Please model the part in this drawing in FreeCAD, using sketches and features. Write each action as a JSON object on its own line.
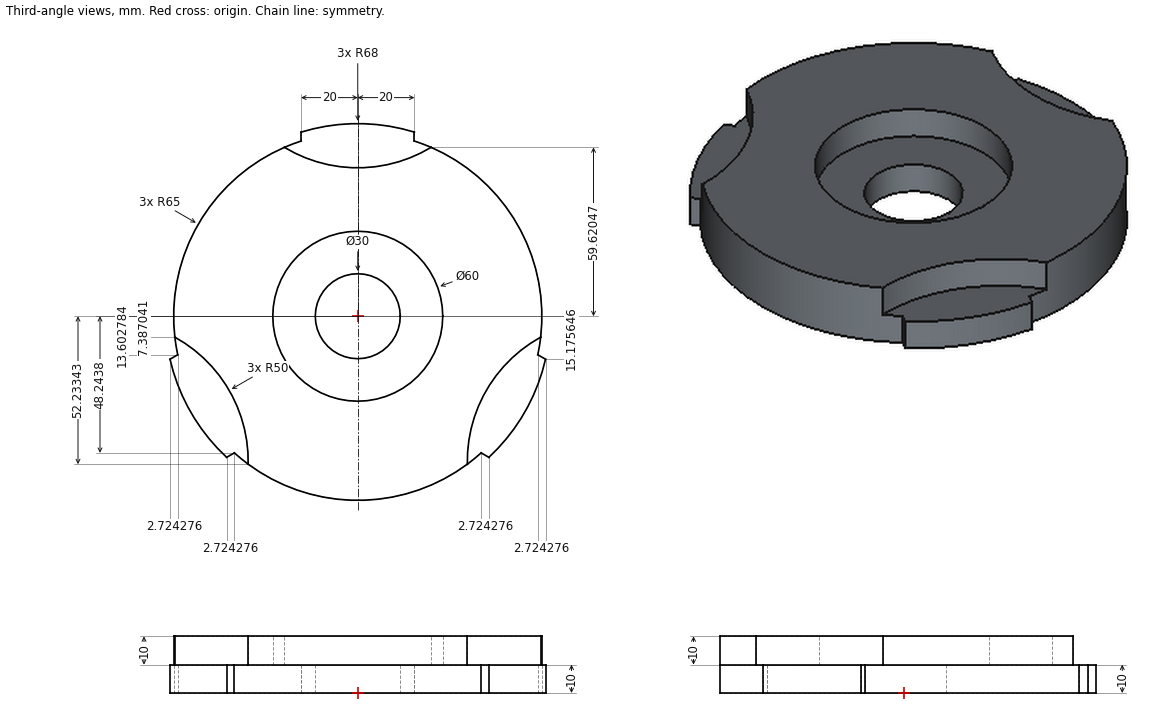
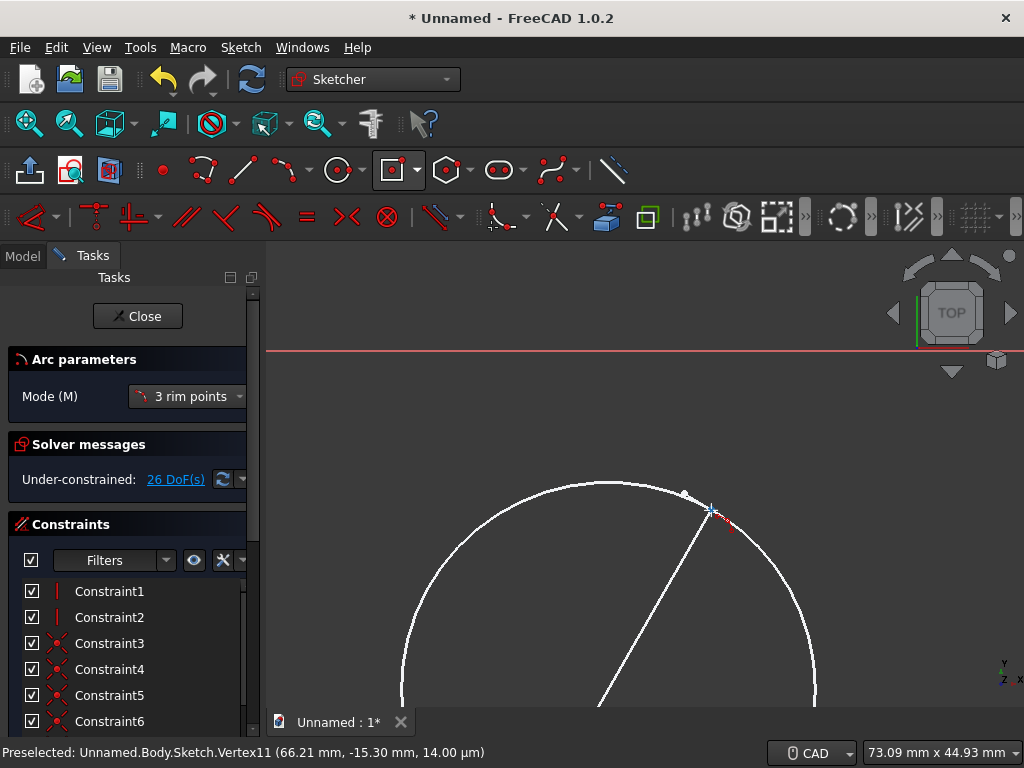
{"action": "scroll", "coordinate": [716, 509], "scroll_direction": "down", "scroll_amount": 8}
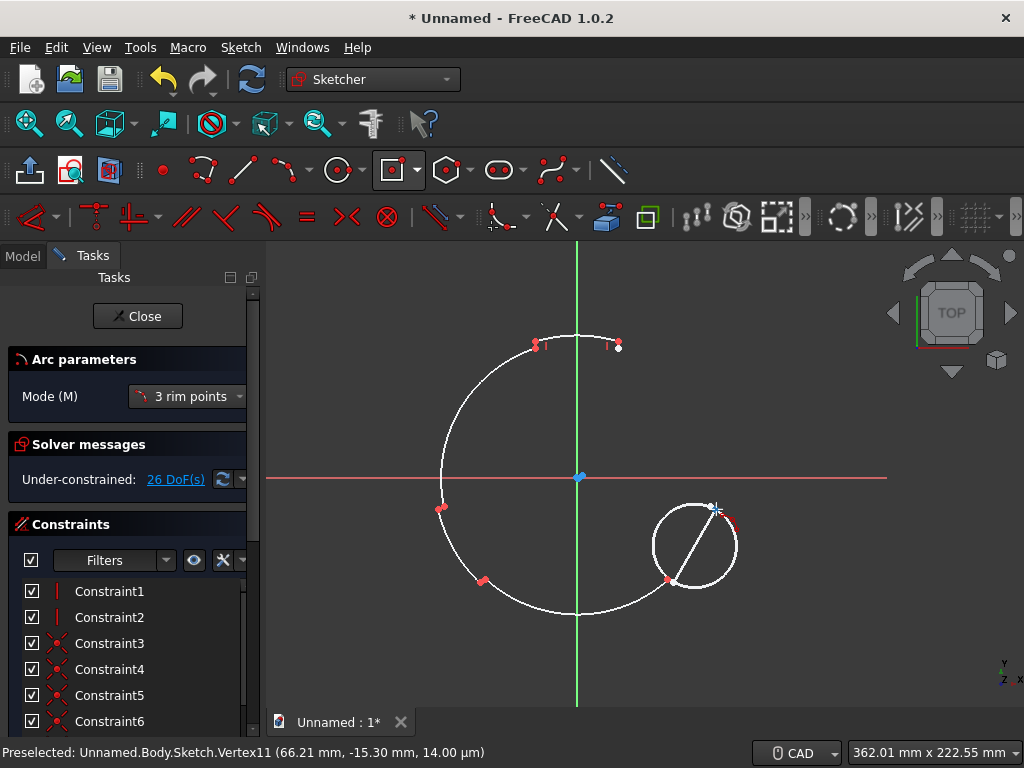
{"action": "scroll", "coordinate": [700, 549], "scroll_direction": "up", "scroll_amount": 5}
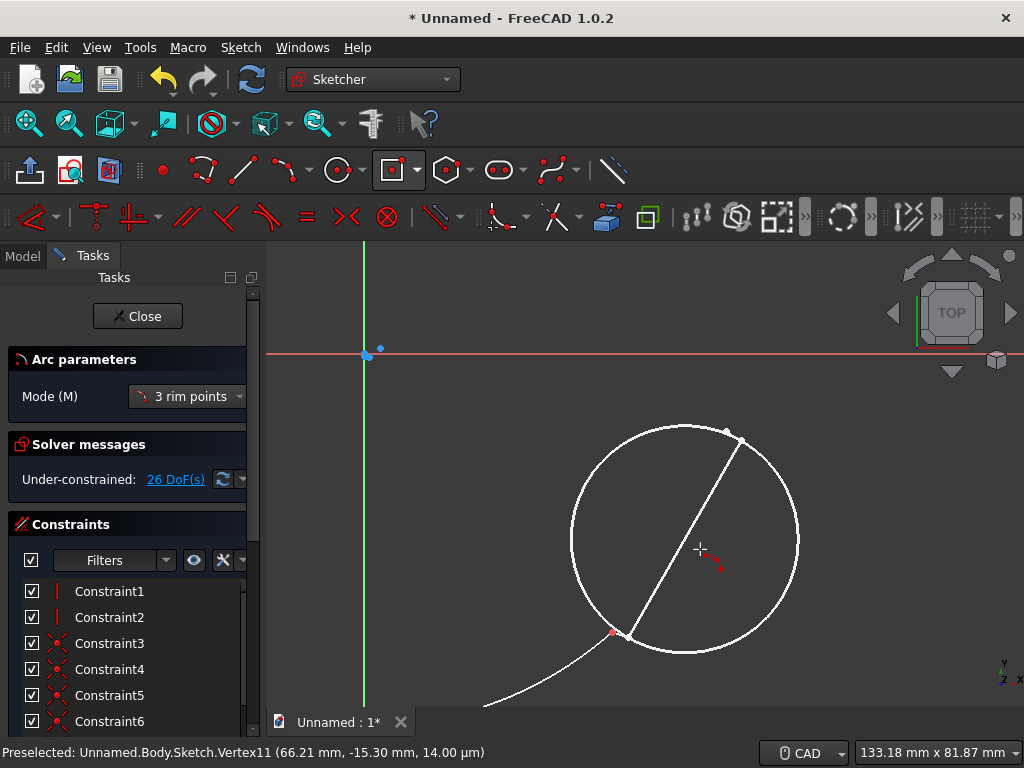
{"action": "left_click", "coordinate": [700, 547]}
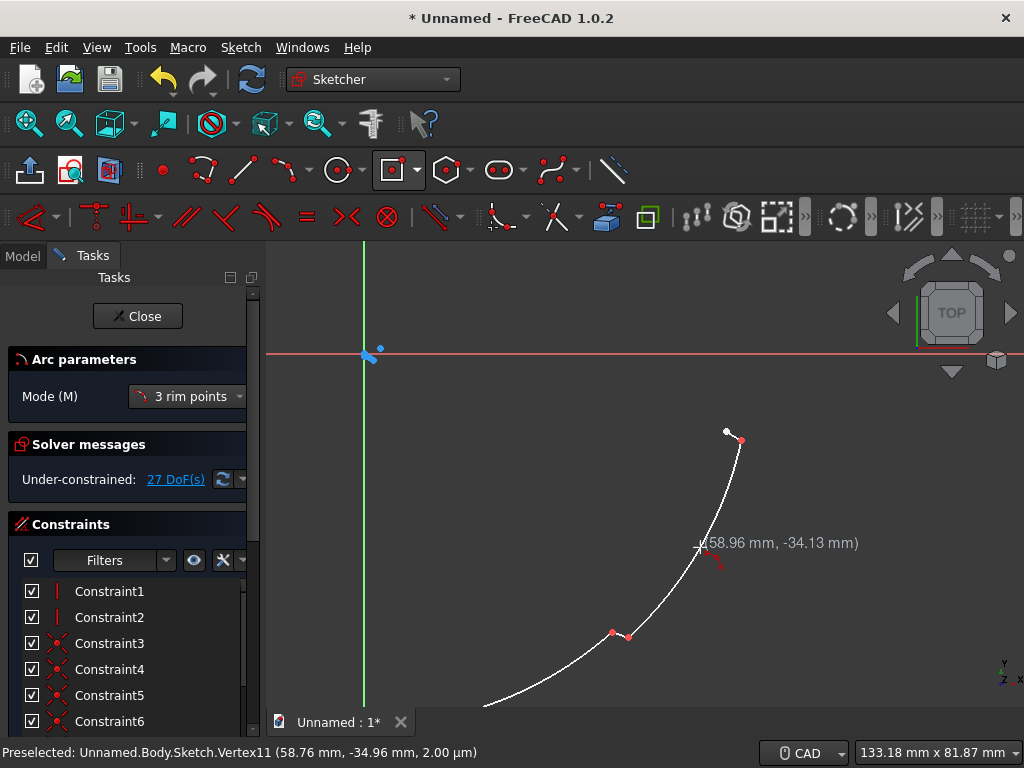
{"action": "scroll", "coordinate": [726, 431], "scroll_direction": "up", "scroll_amount": 3}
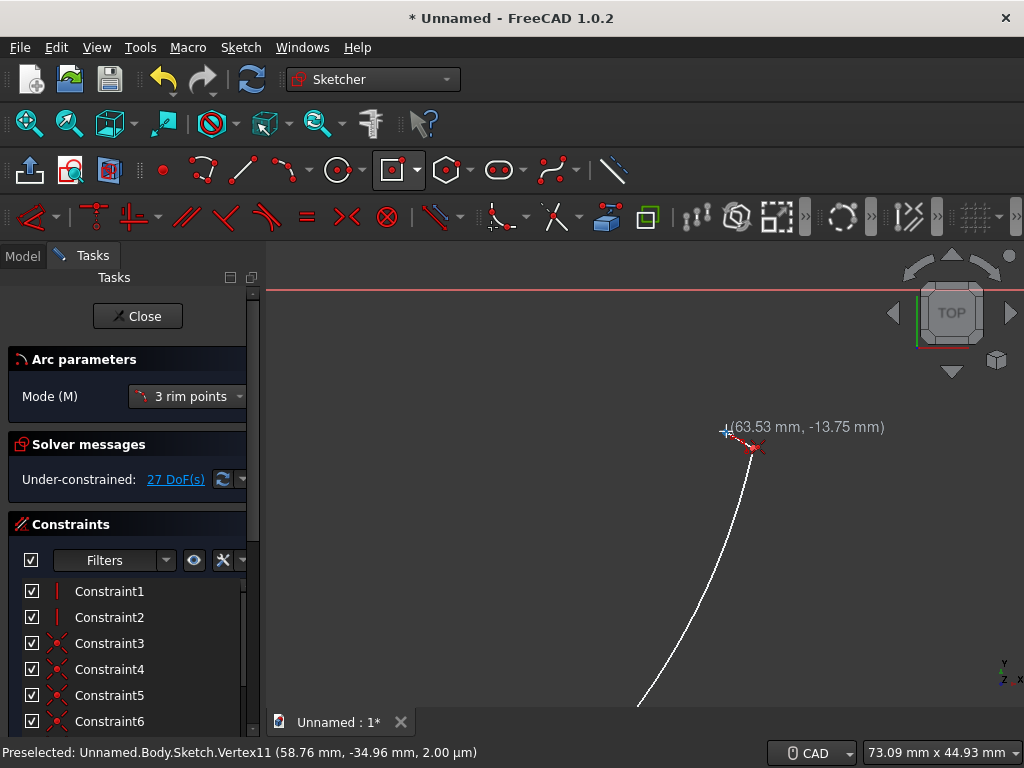
{"action": "left_click", "coordinate": [726, 432]}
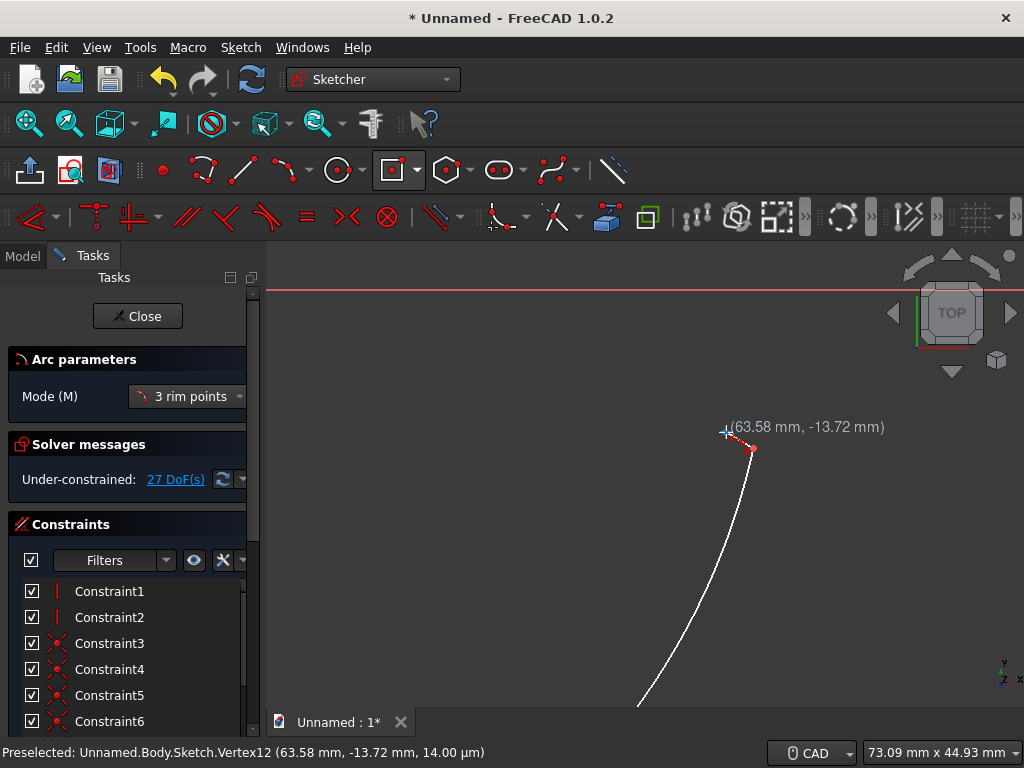
{"action": "scroll", "coordinate": [705, 525], "scroll_direction": "down", "scroll_amount": 8}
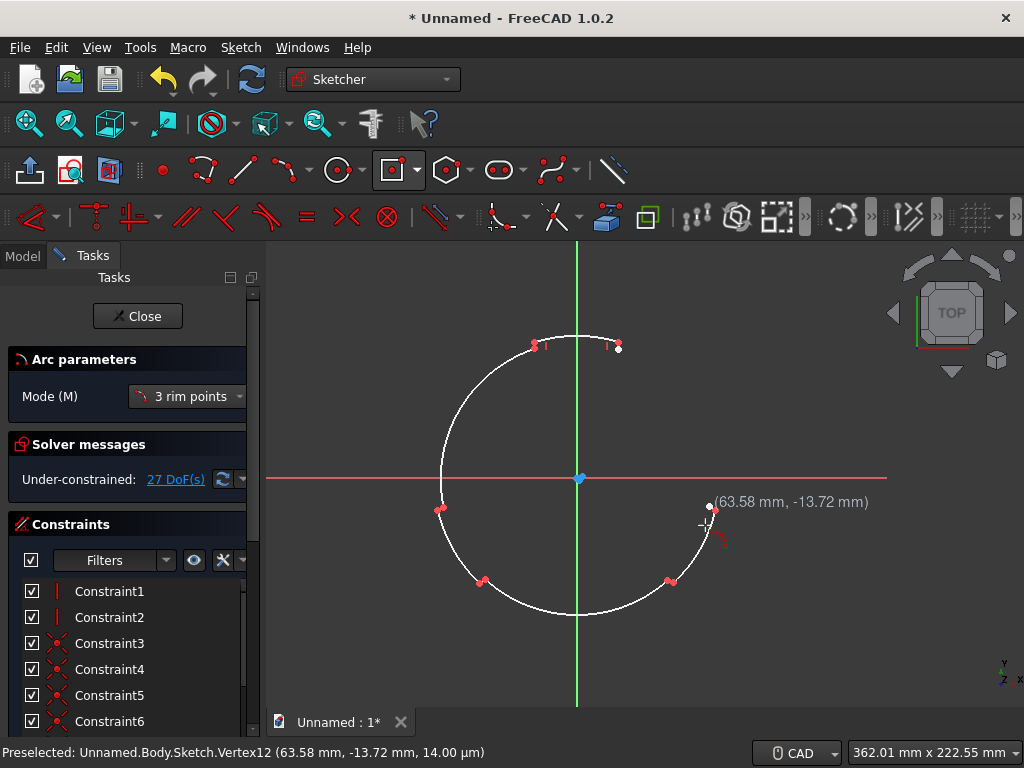
{"action": "scroll", "coordinate": [618, 349], "scroll_direction": "up", "scroll_amount": 8}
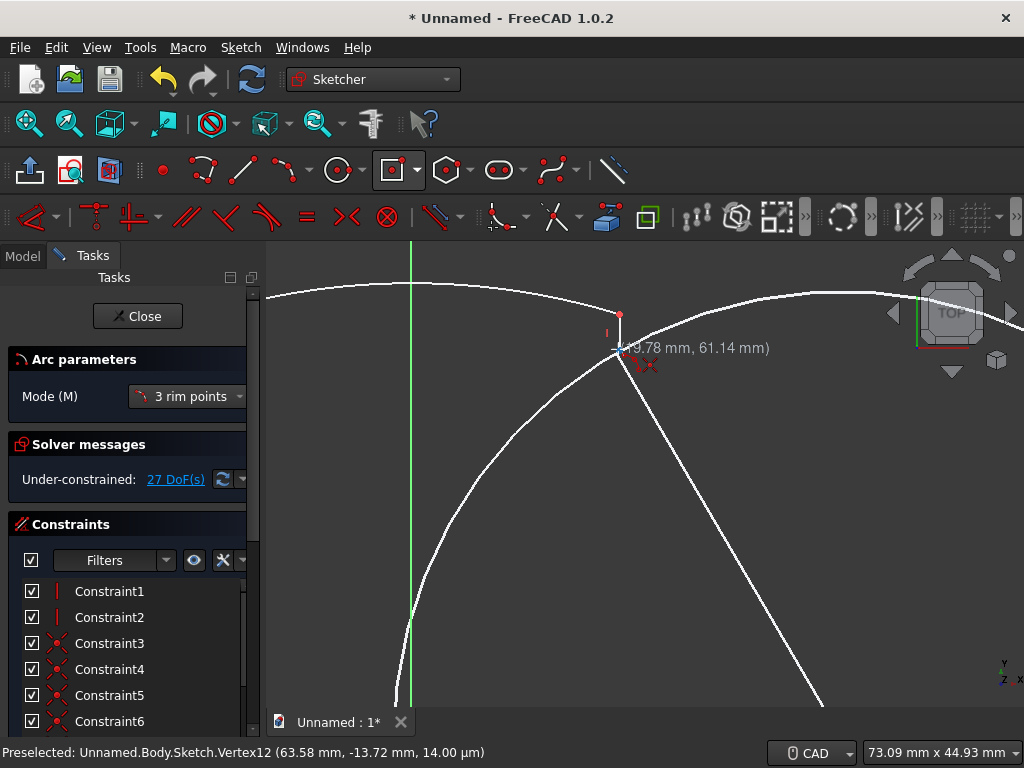
{"action": "left_click", "coordinate": [620, 350]}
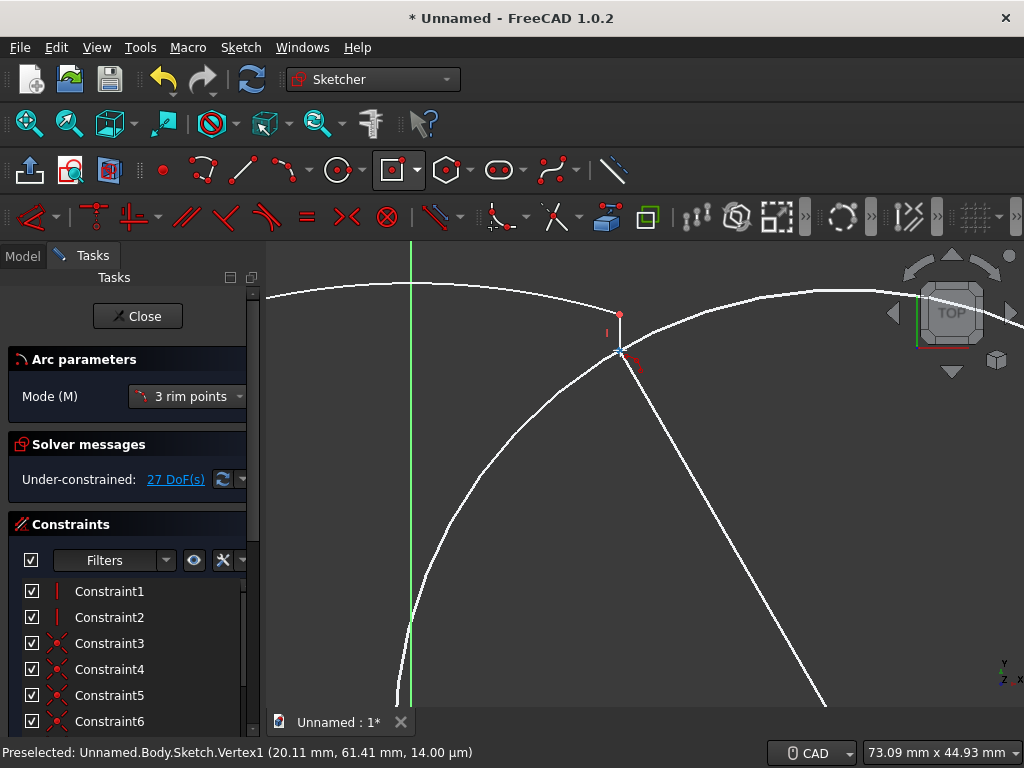
{"action": "scroll", "coordinate": [618, 348], "scroll_direction": "down", "scroll_amount": 8}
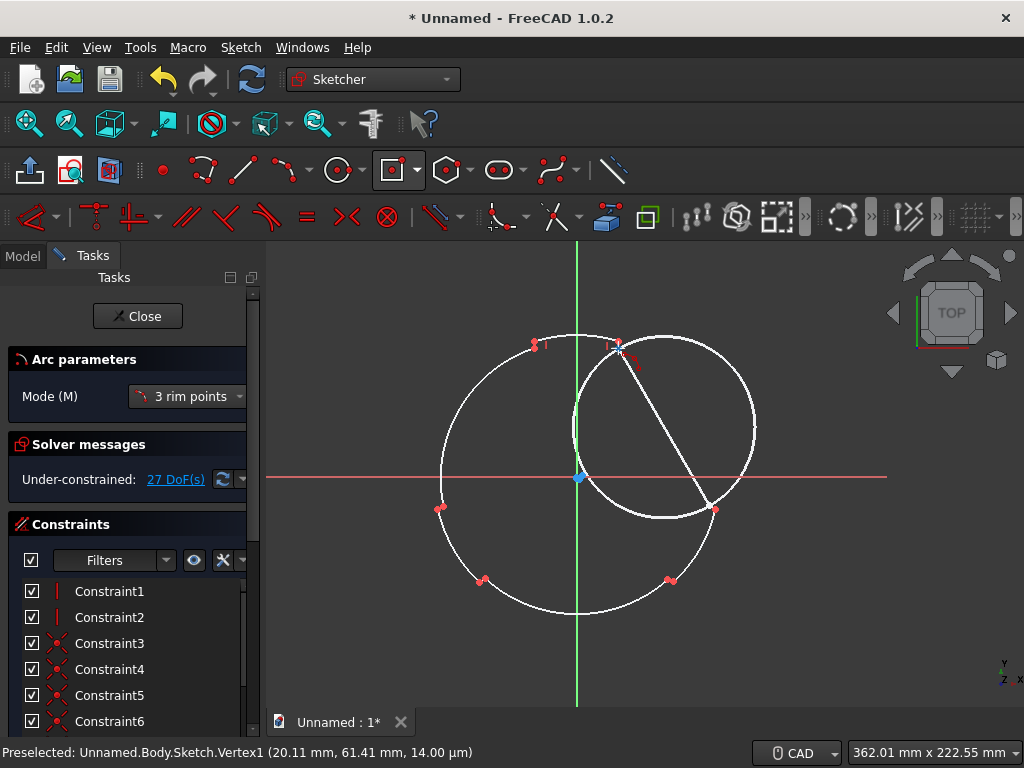
{"action": "left_click", "coordinate": [694, 409]}
{"action": "key", "text": "Escape"}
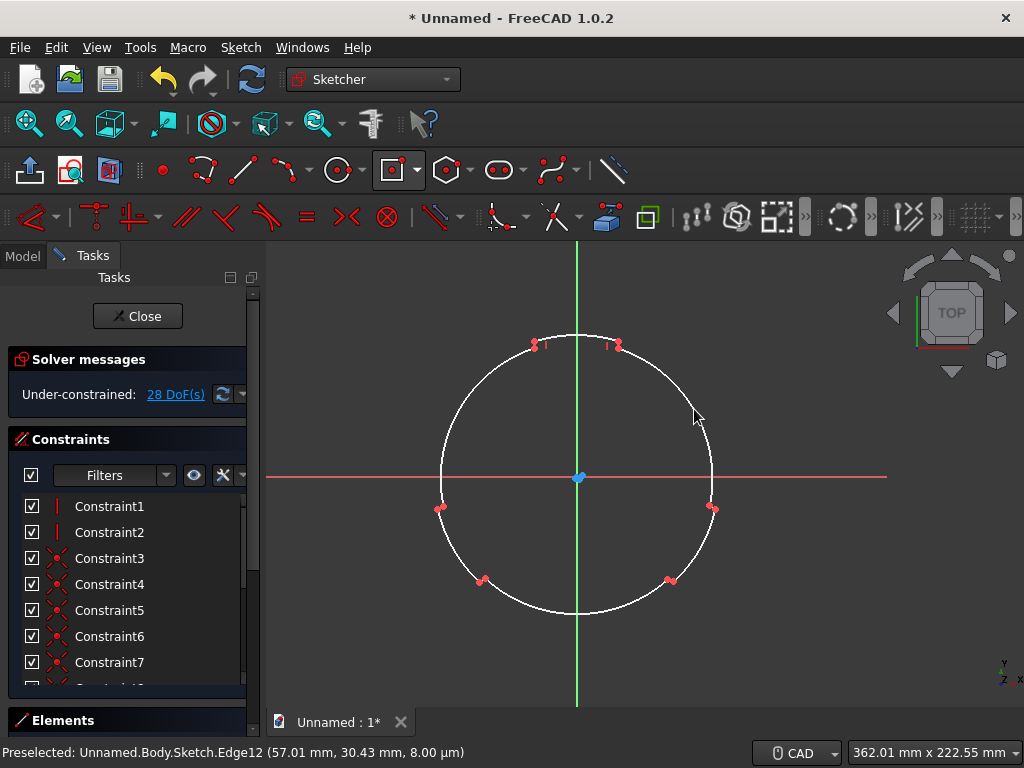
{"action": "left_click", "coordinate": [594, 336]}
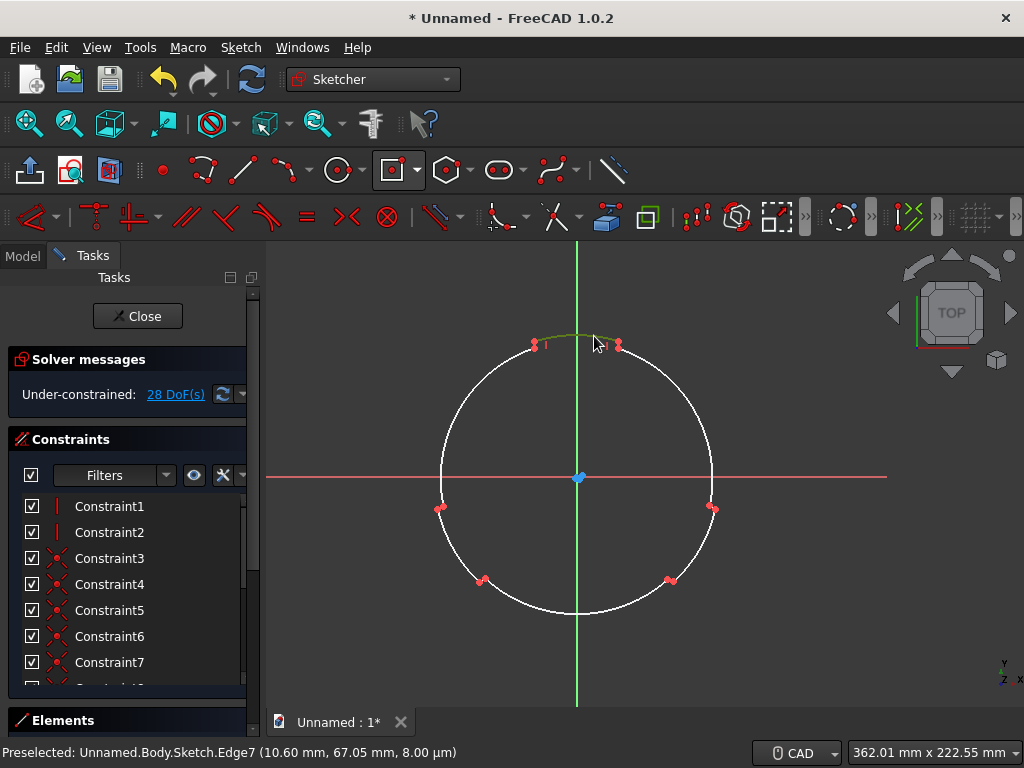
{"action": "left_click", "coordinate": [484, 379]}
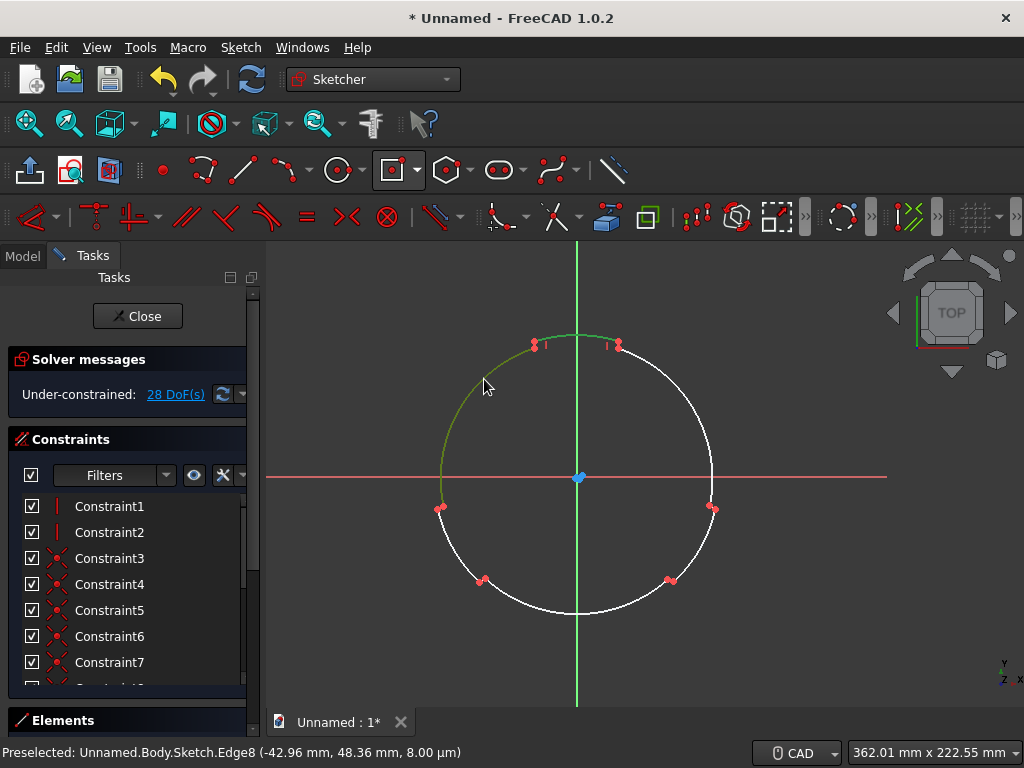
{"action": "left_click", "coordinate": [94, 218]}